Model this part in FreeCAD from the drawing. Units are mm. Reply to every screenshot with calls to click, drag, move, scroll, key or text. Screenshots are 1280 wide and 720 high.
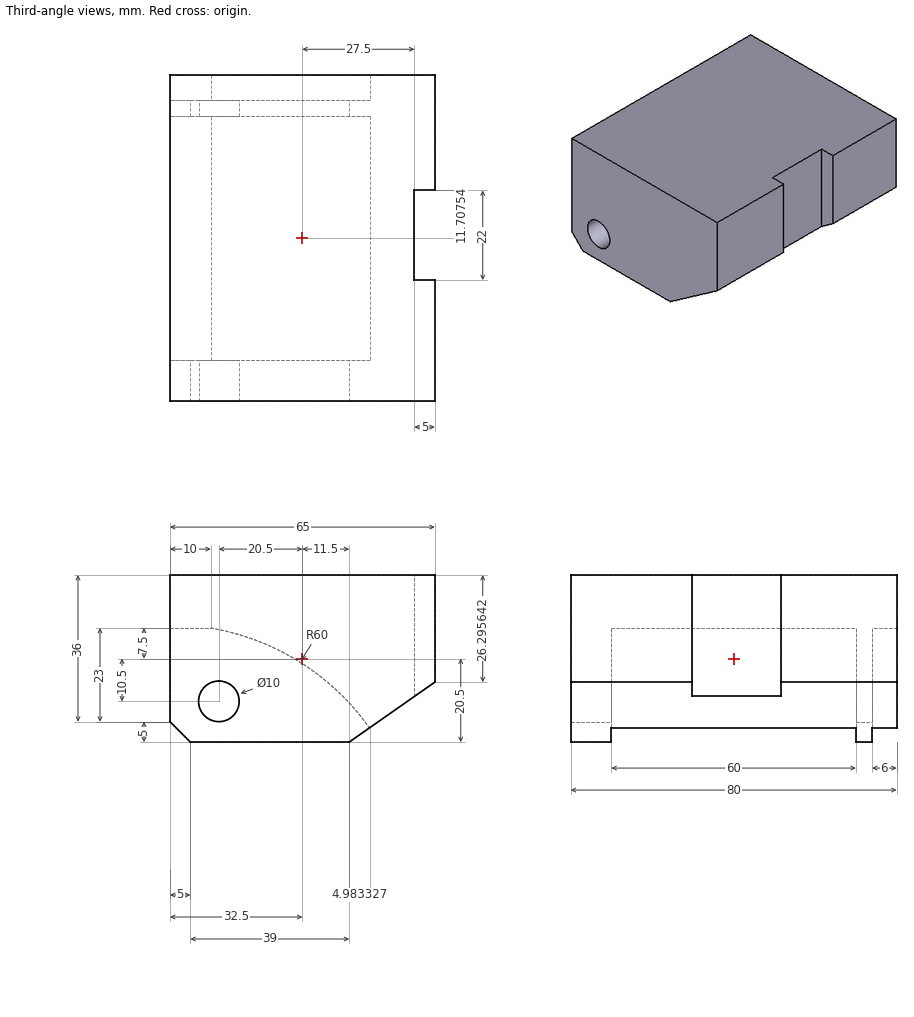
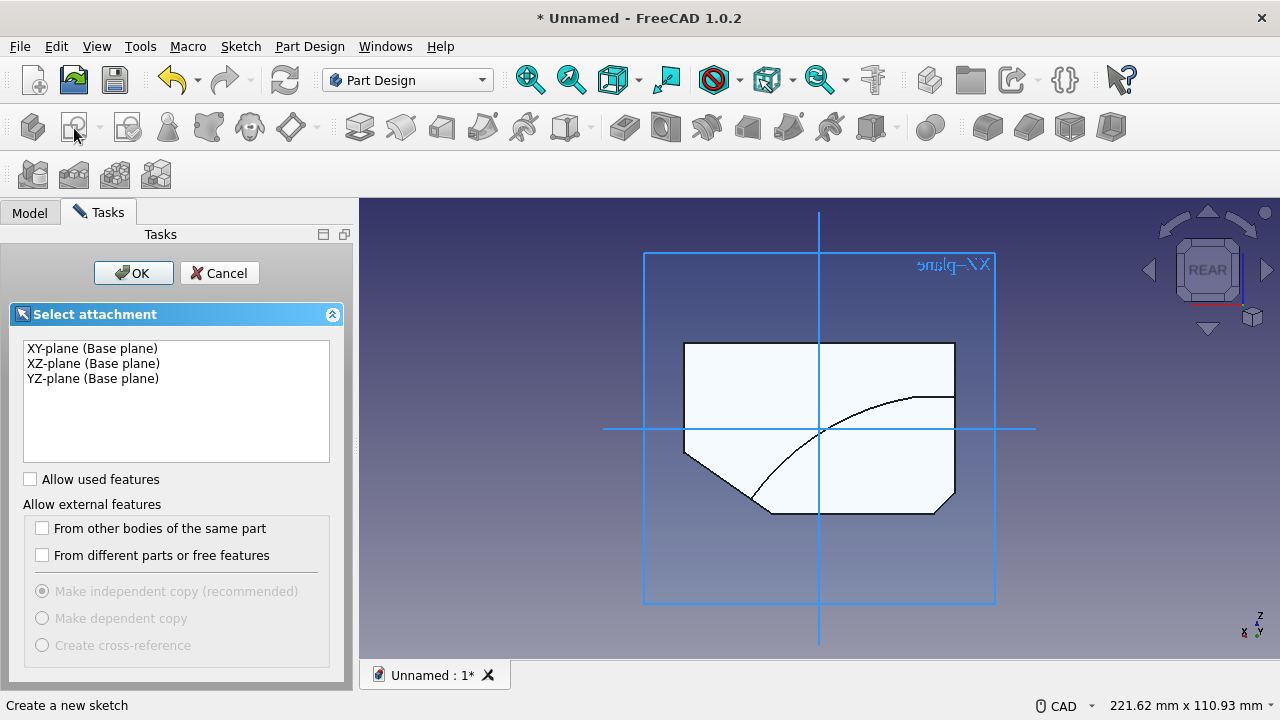
click(84, 364)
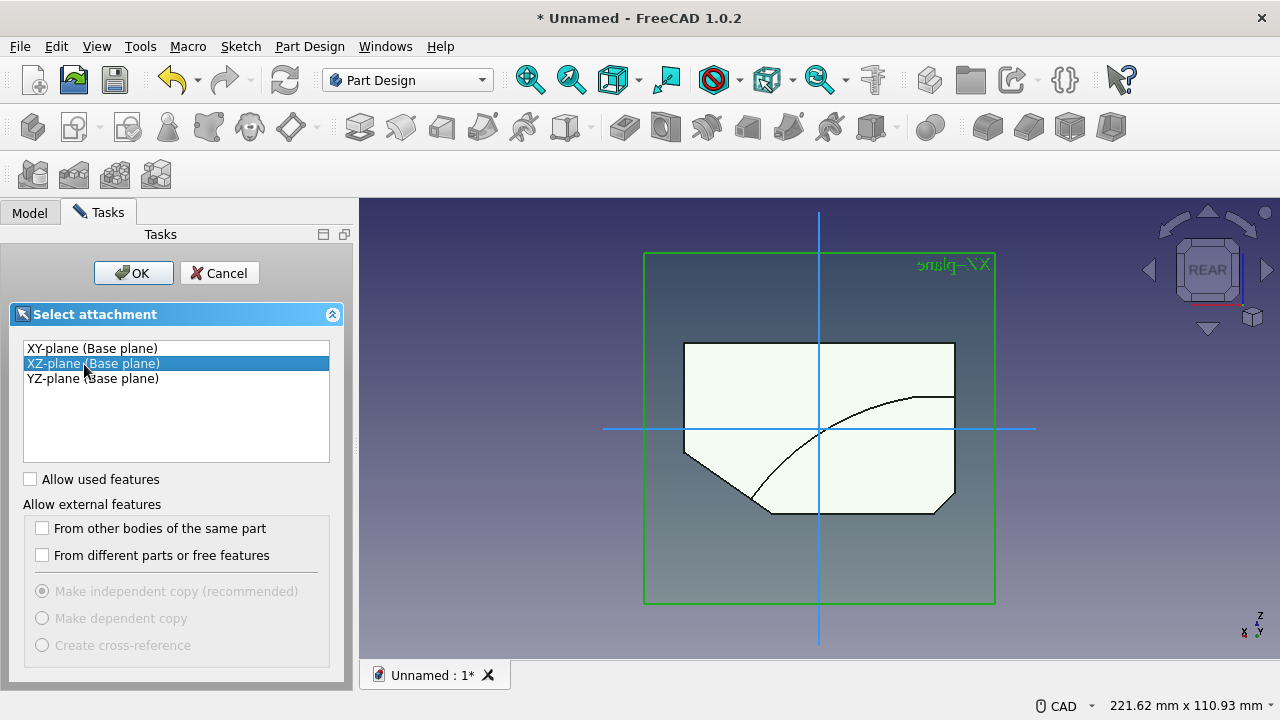
click(134, 273)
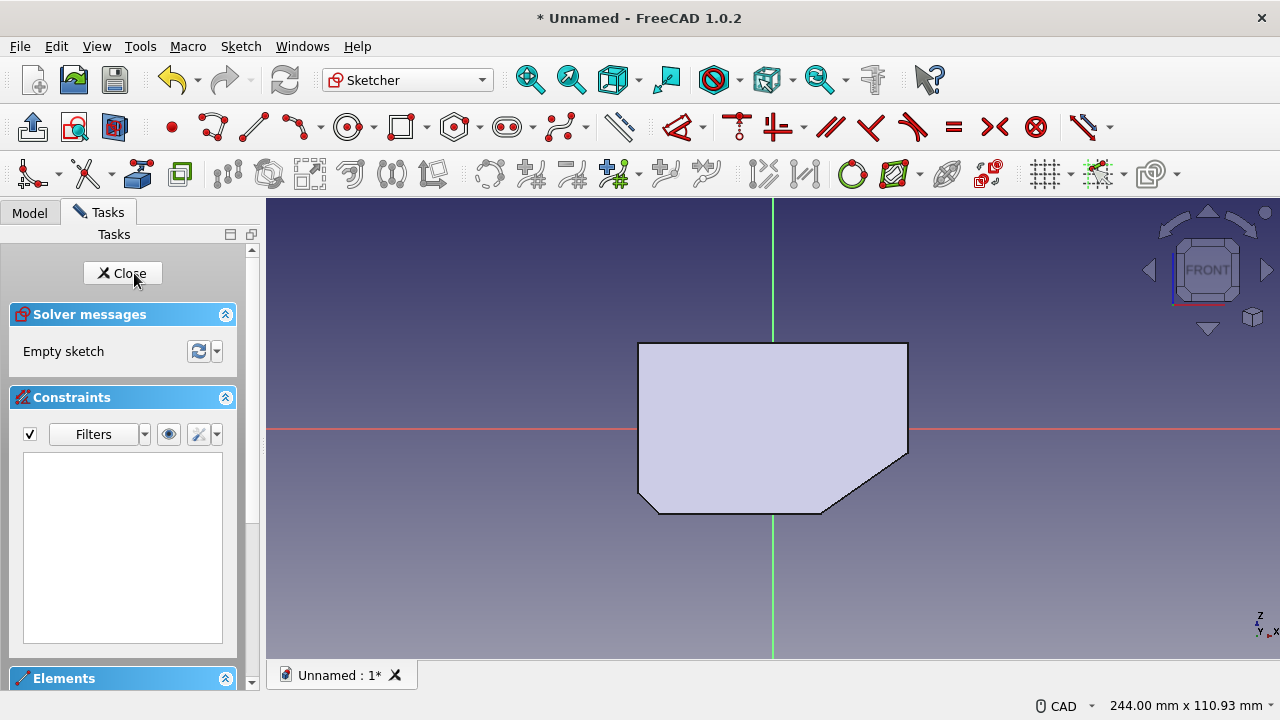
key(q)
key(s)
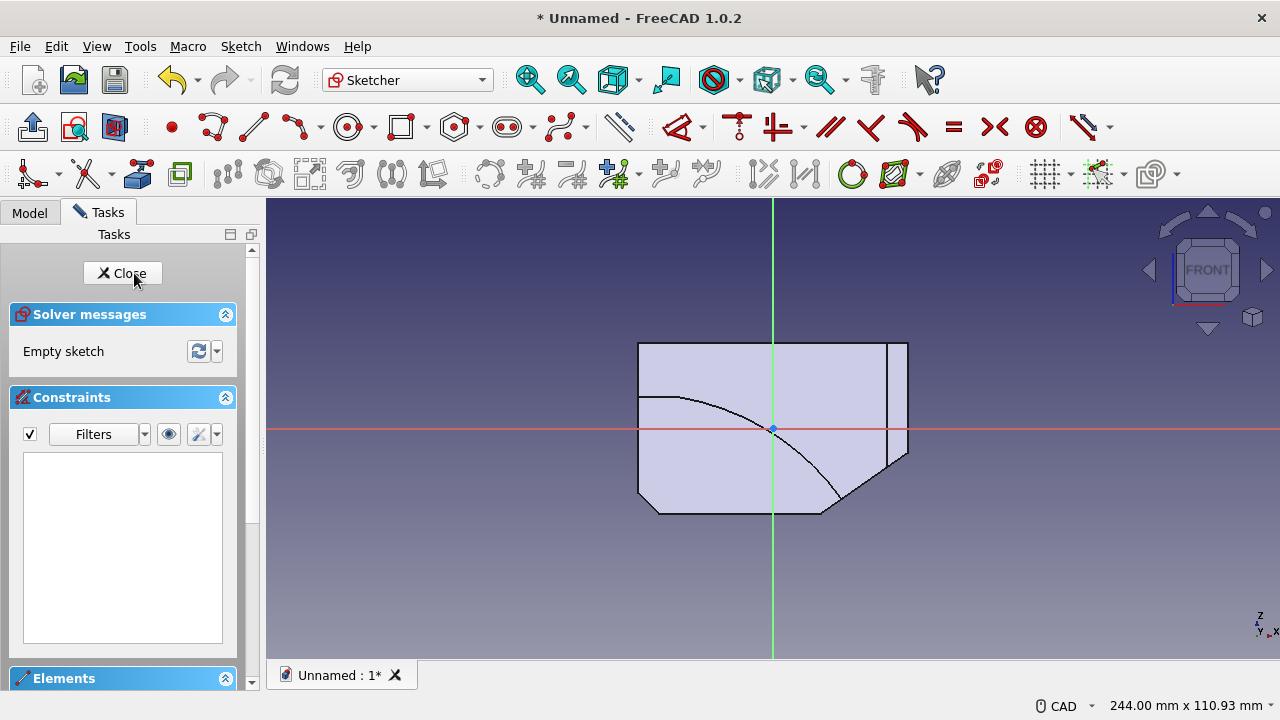
scroll(768, 478, up, 4)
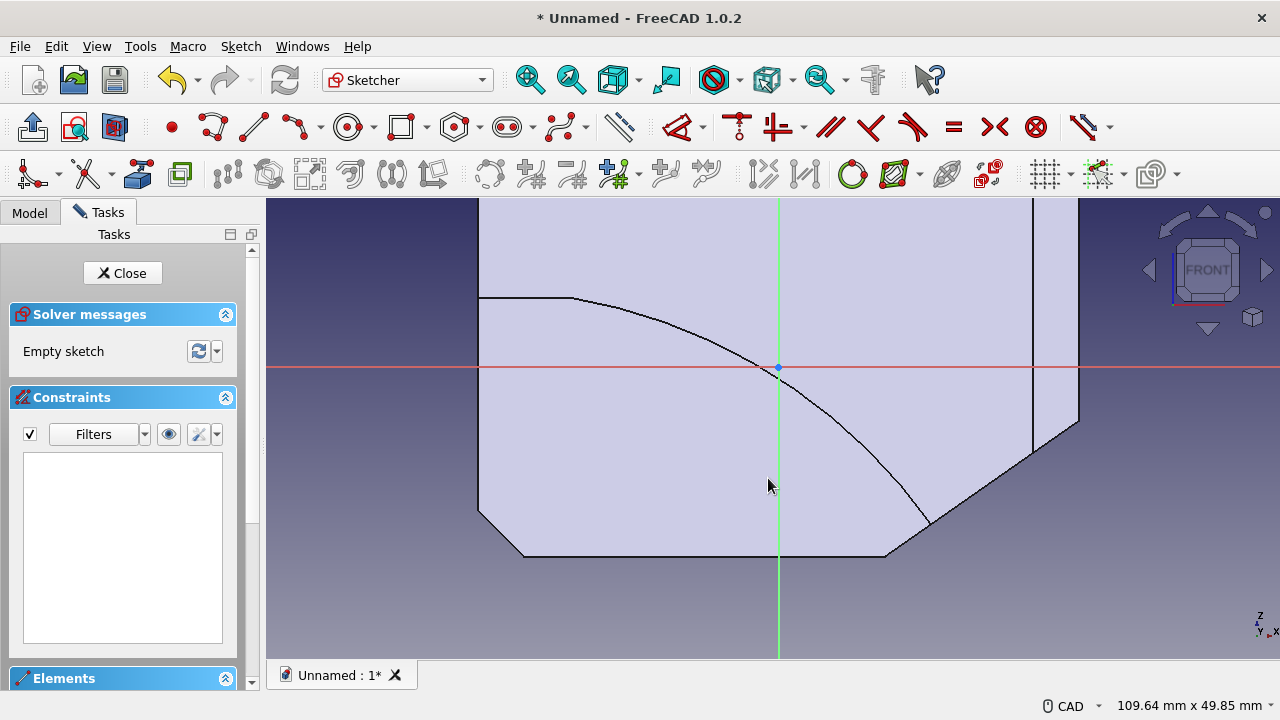
key(g)
key(m)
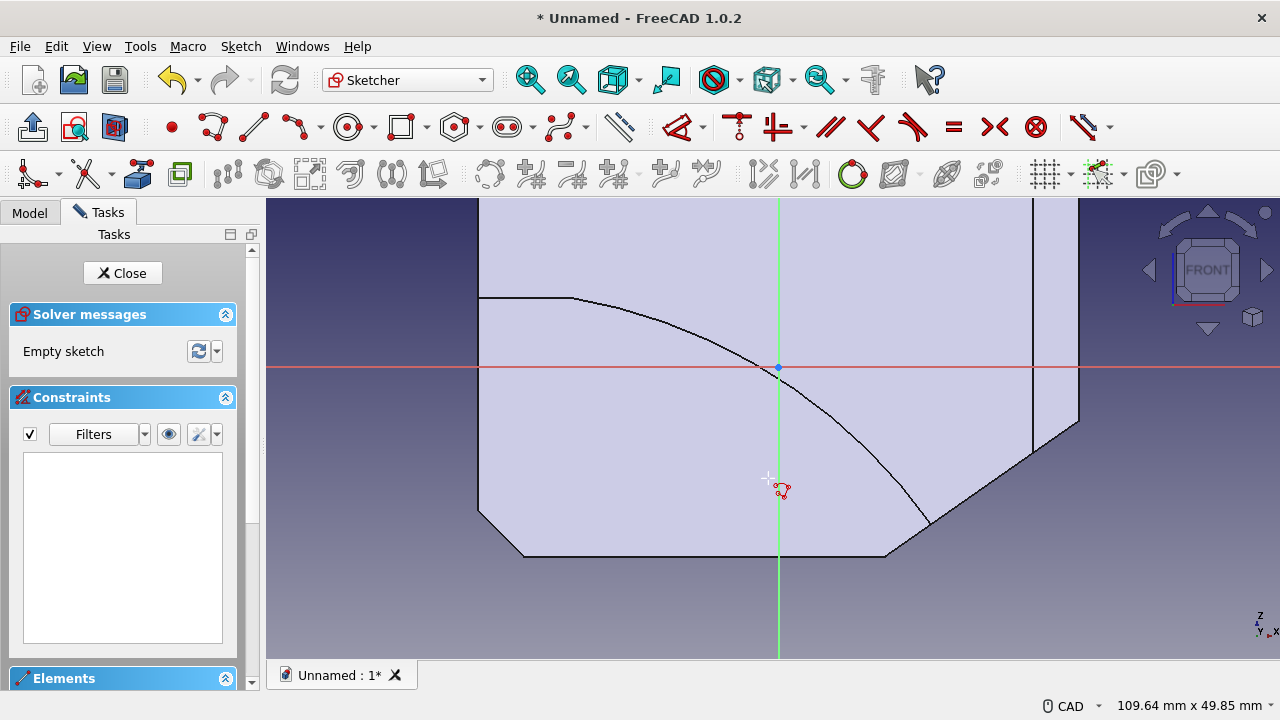
click(931, 524)
click(885, 557)
click(524, 557)
click(478, 510)
click(478, 298)
click(570, 298)
right_click(570, 298)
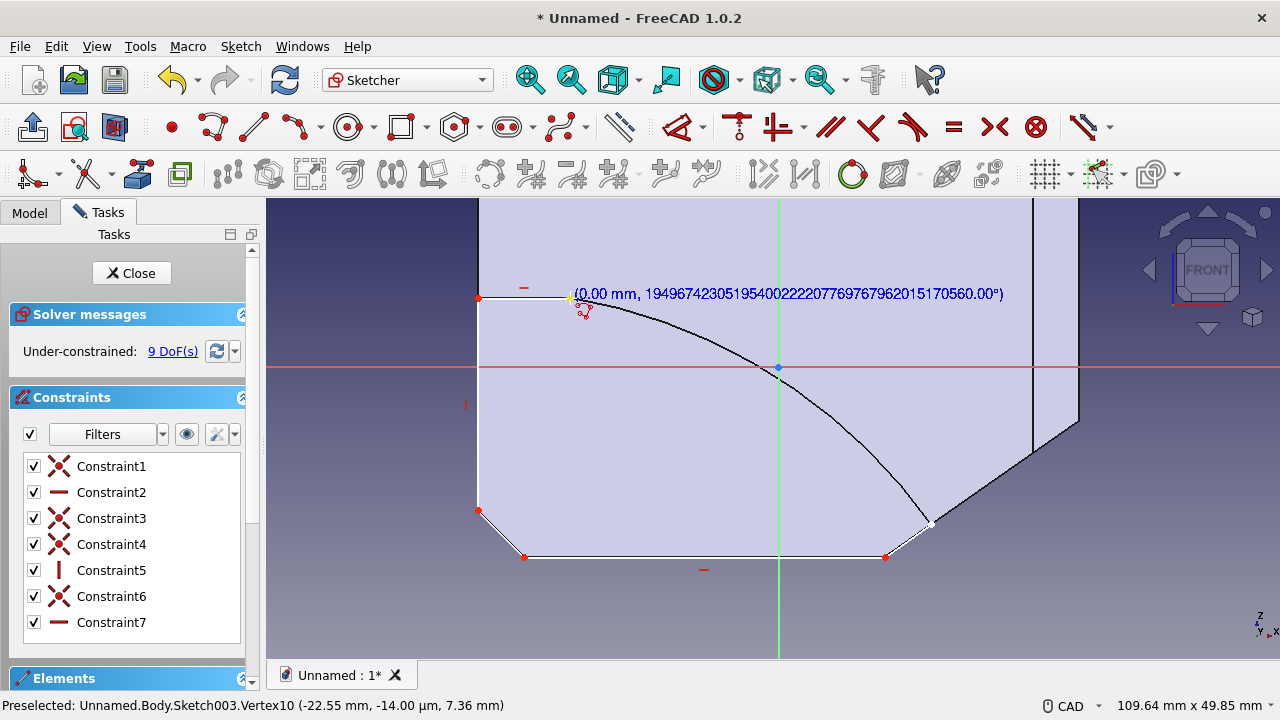
click(294, 128)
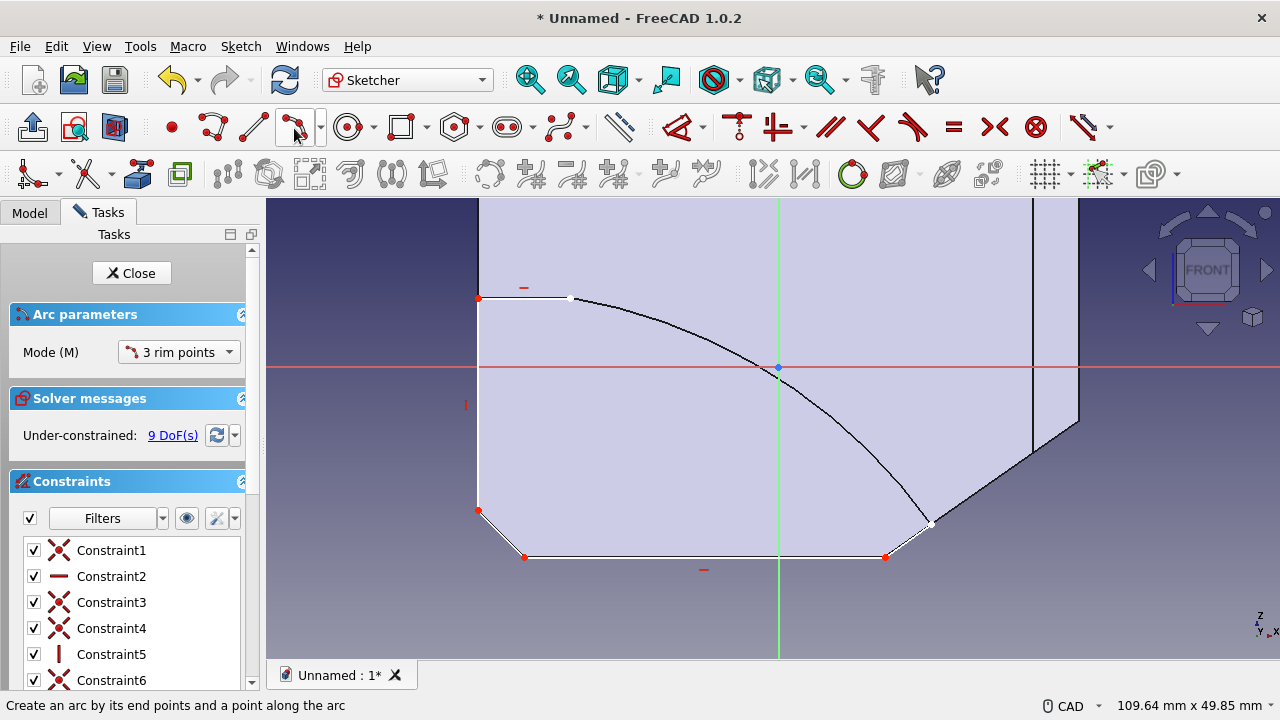
click(570, 299)
click(931, 525)
click(809, 400)
key(Escape)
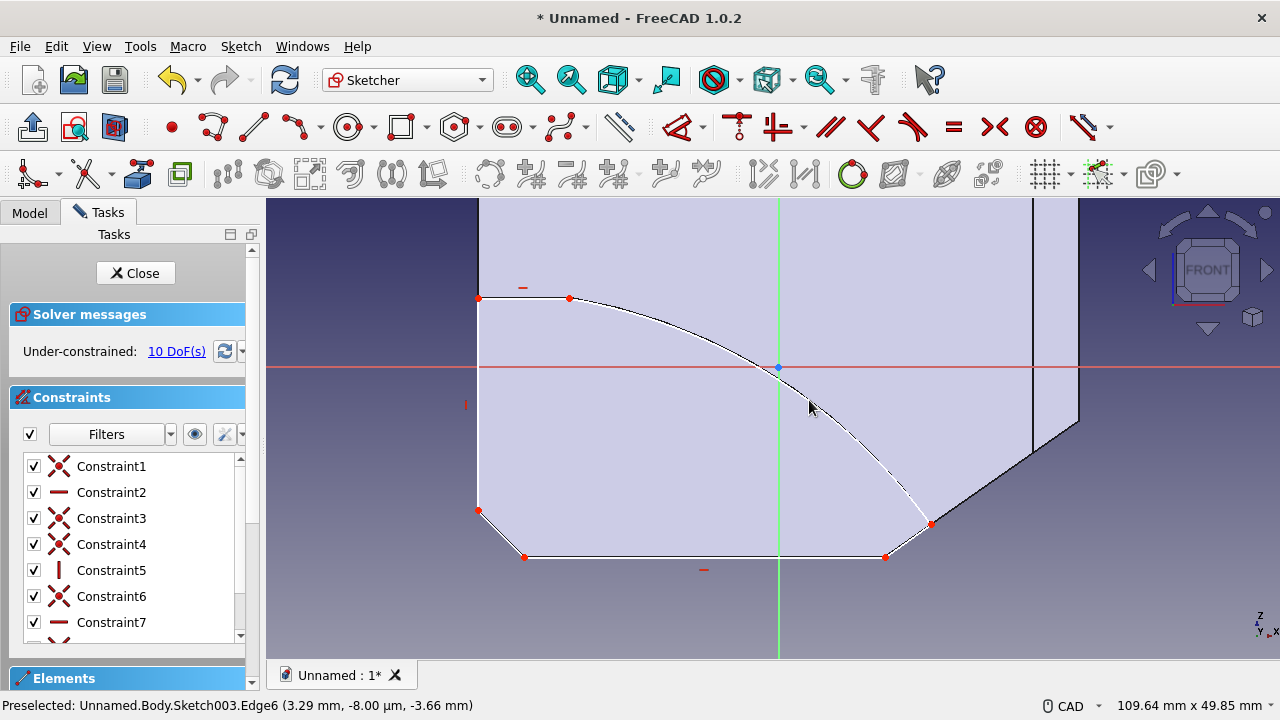
click(676, 128)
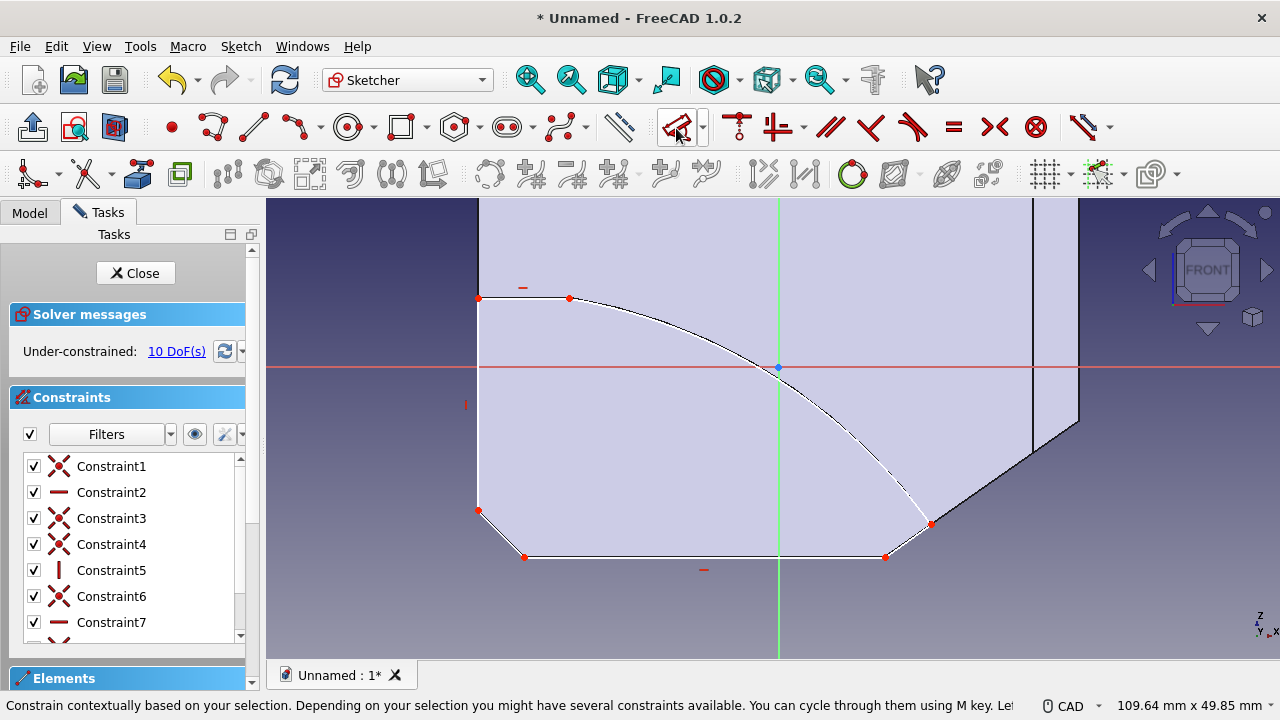
click(843, 428)
click(864, 404)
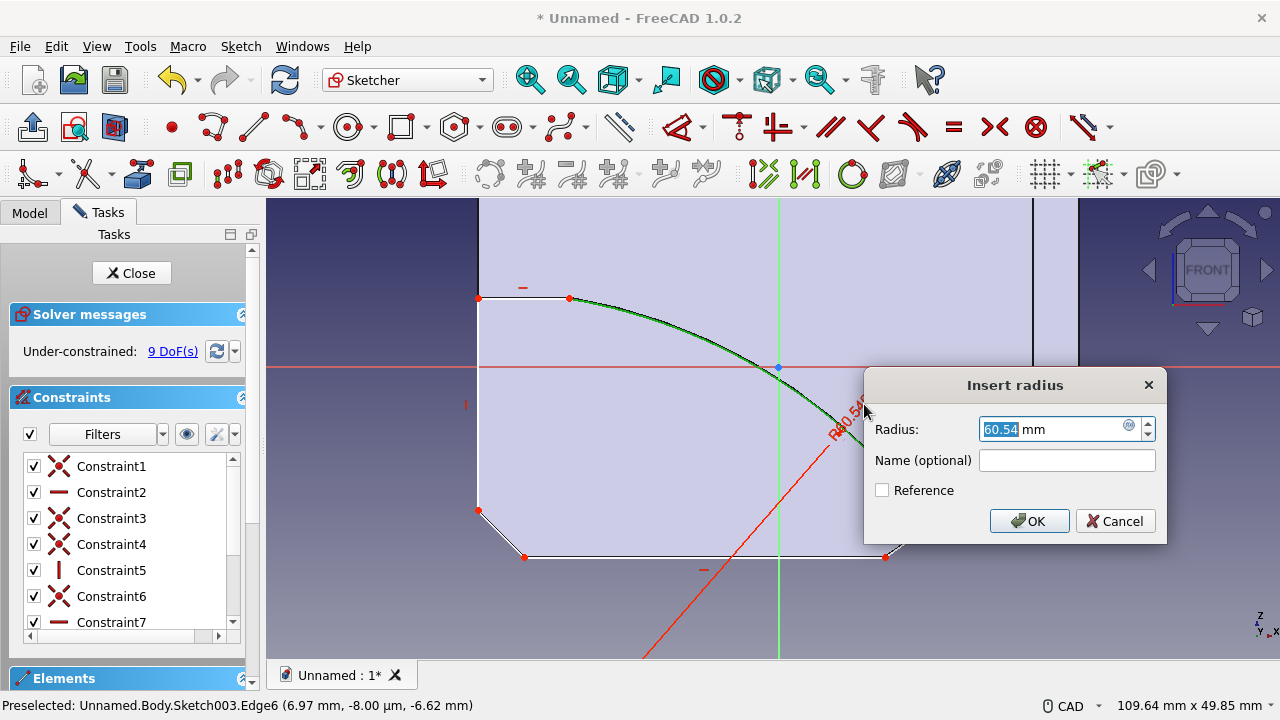
text(60)
key(Return)